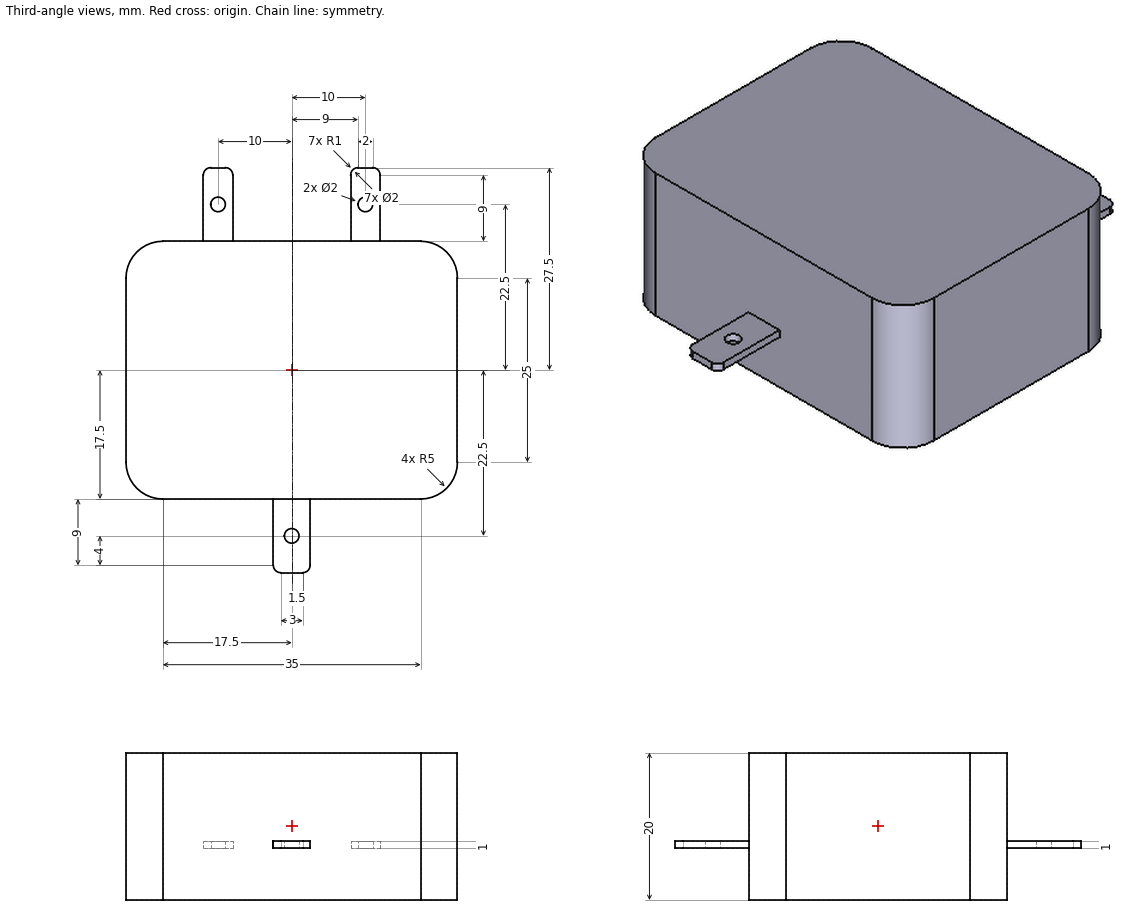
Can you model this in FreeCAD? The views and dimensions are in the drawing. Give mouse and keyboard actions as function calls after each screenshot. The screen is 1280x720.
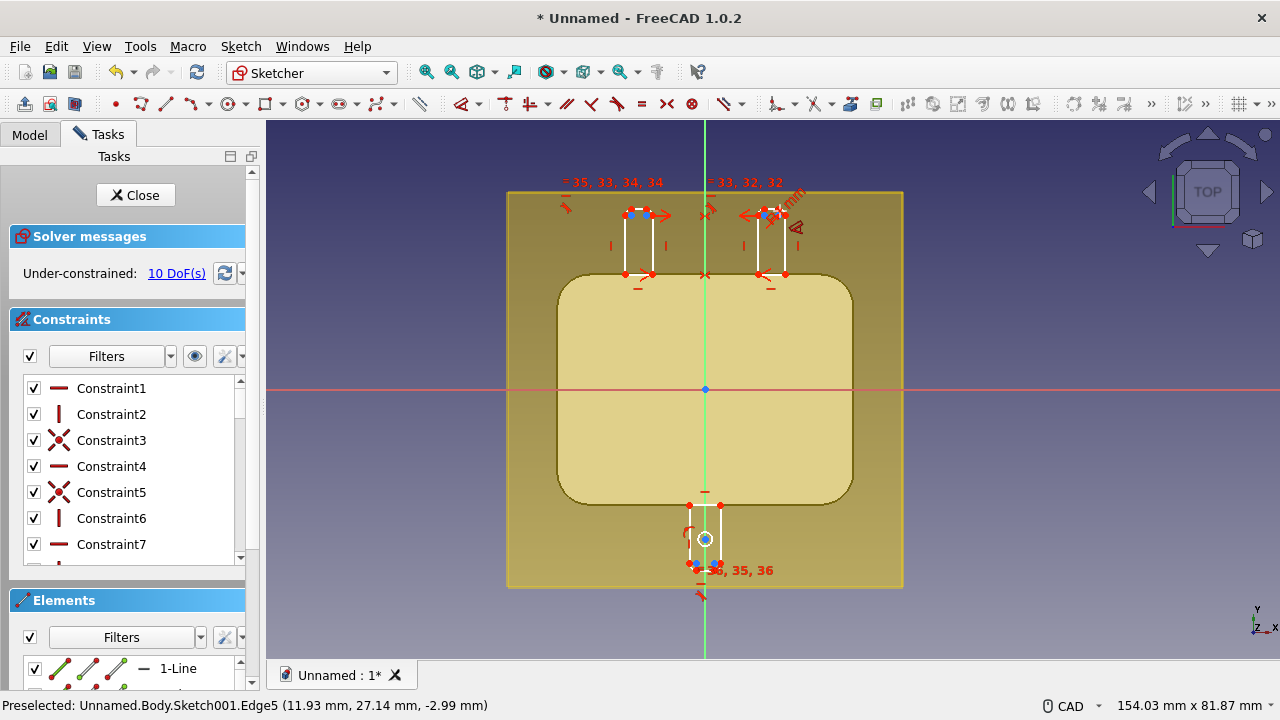
scroll(710, 534, up, 6)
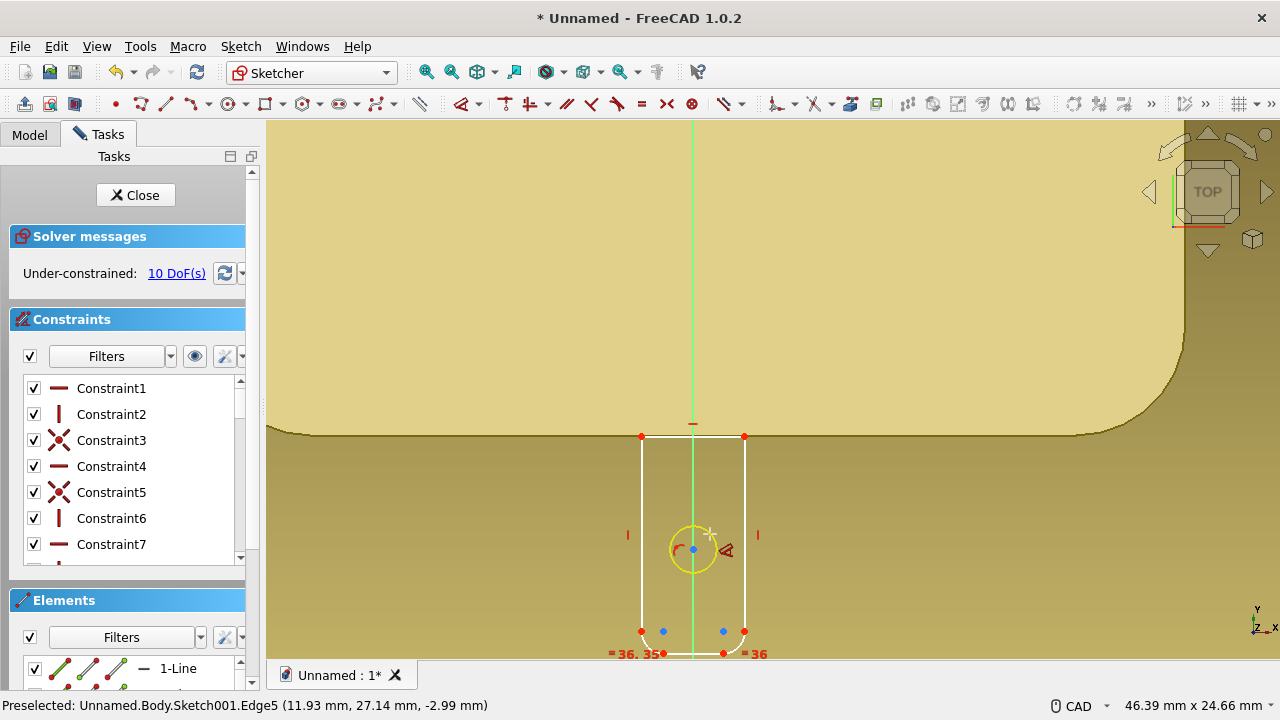
click(710, 533)
click(709, 496)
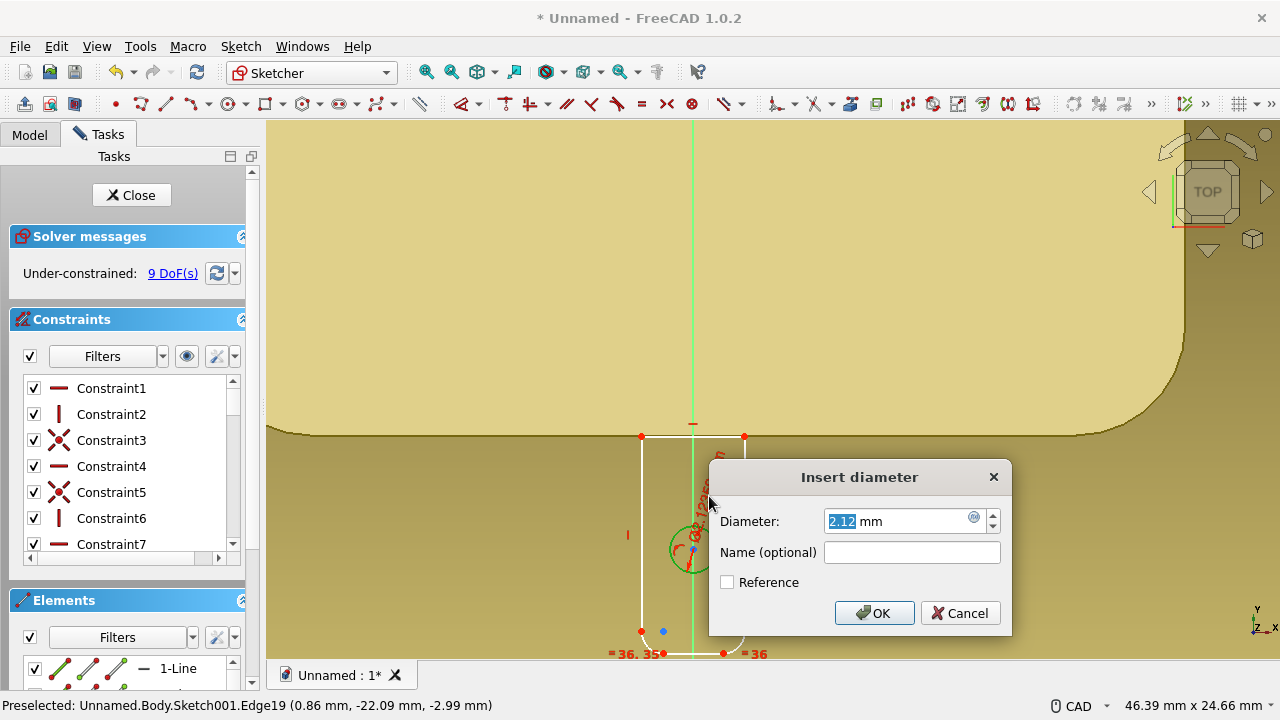
text(2)
key(Return)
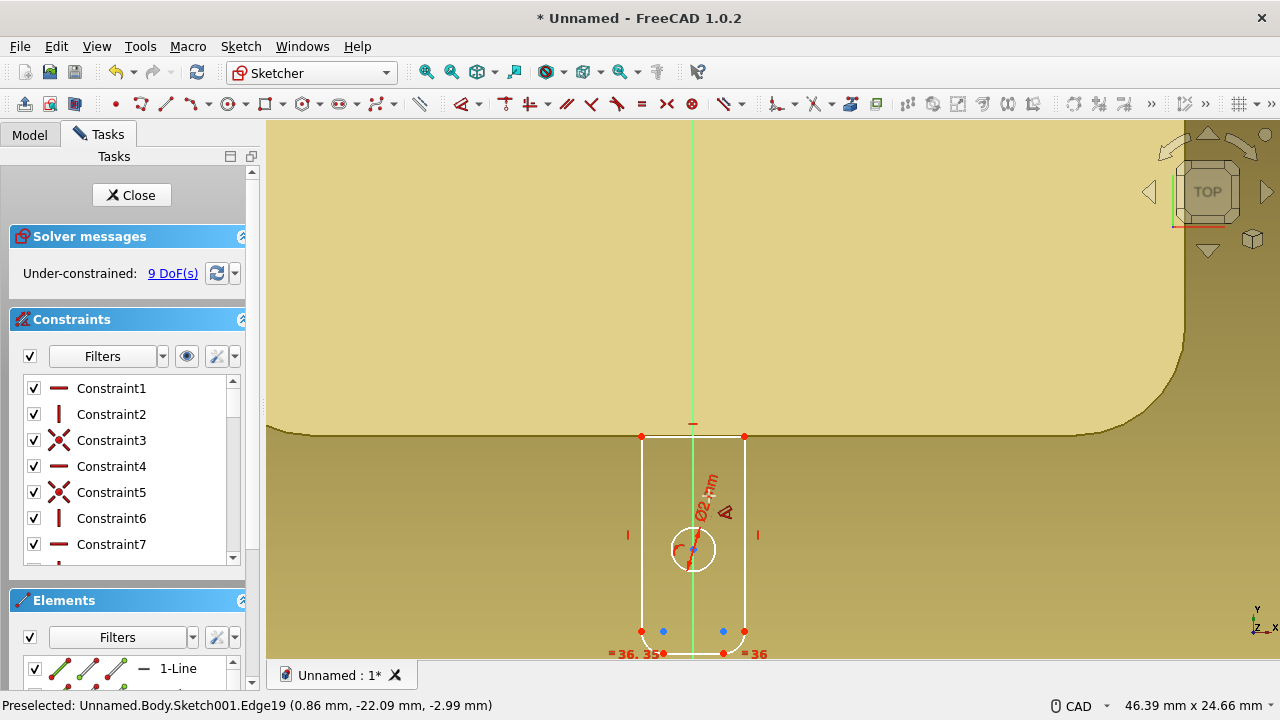
scroll(709, 535, down, 6)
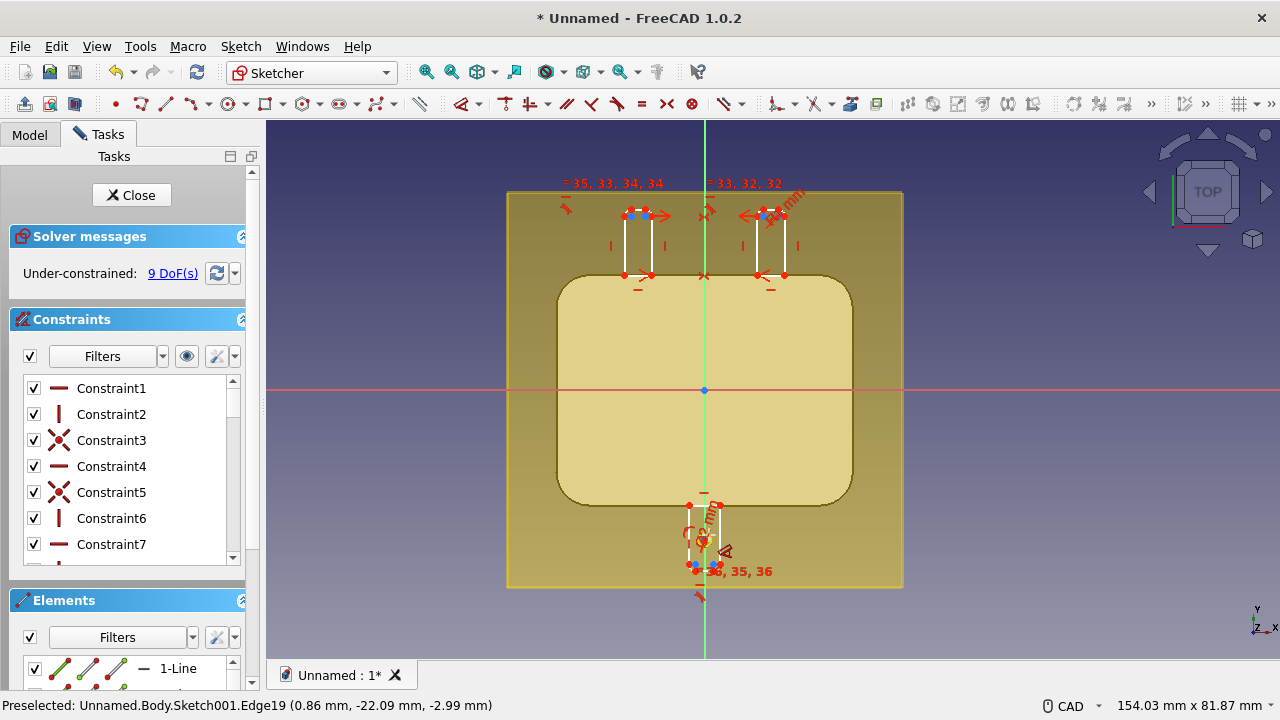
scroll(768, 210, up, 6)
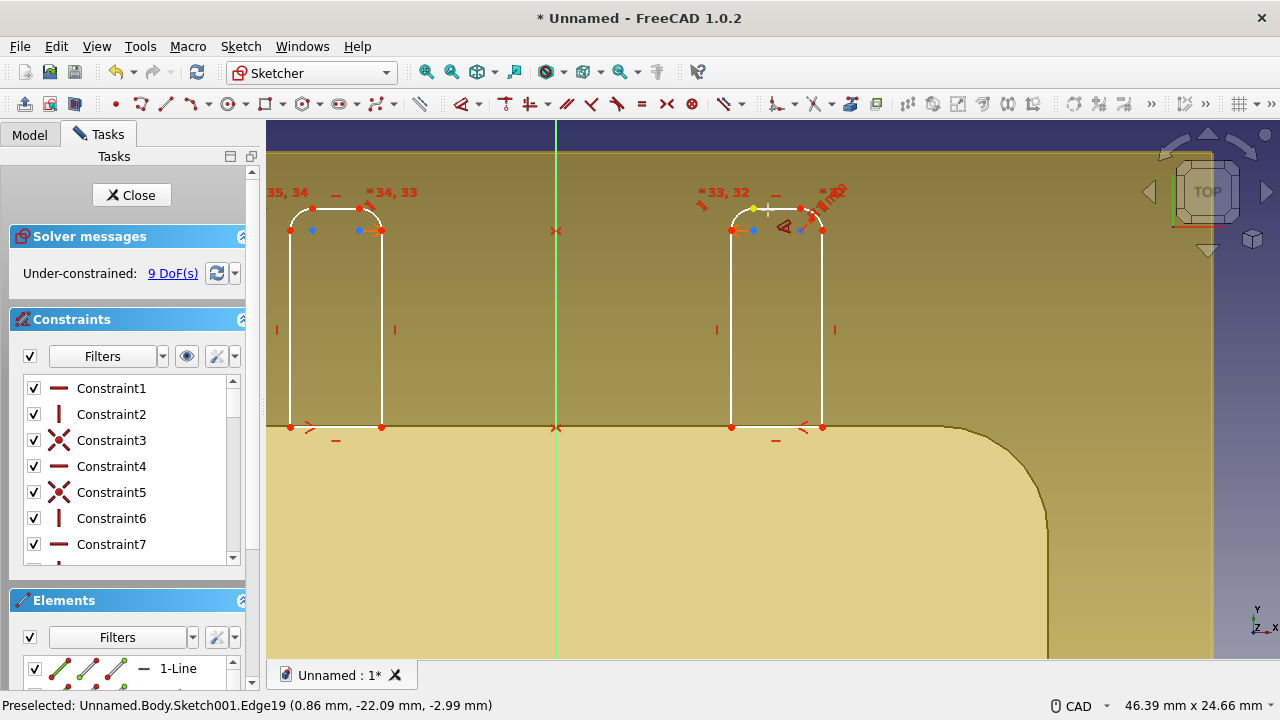
click(767, 209)
click(777, 175)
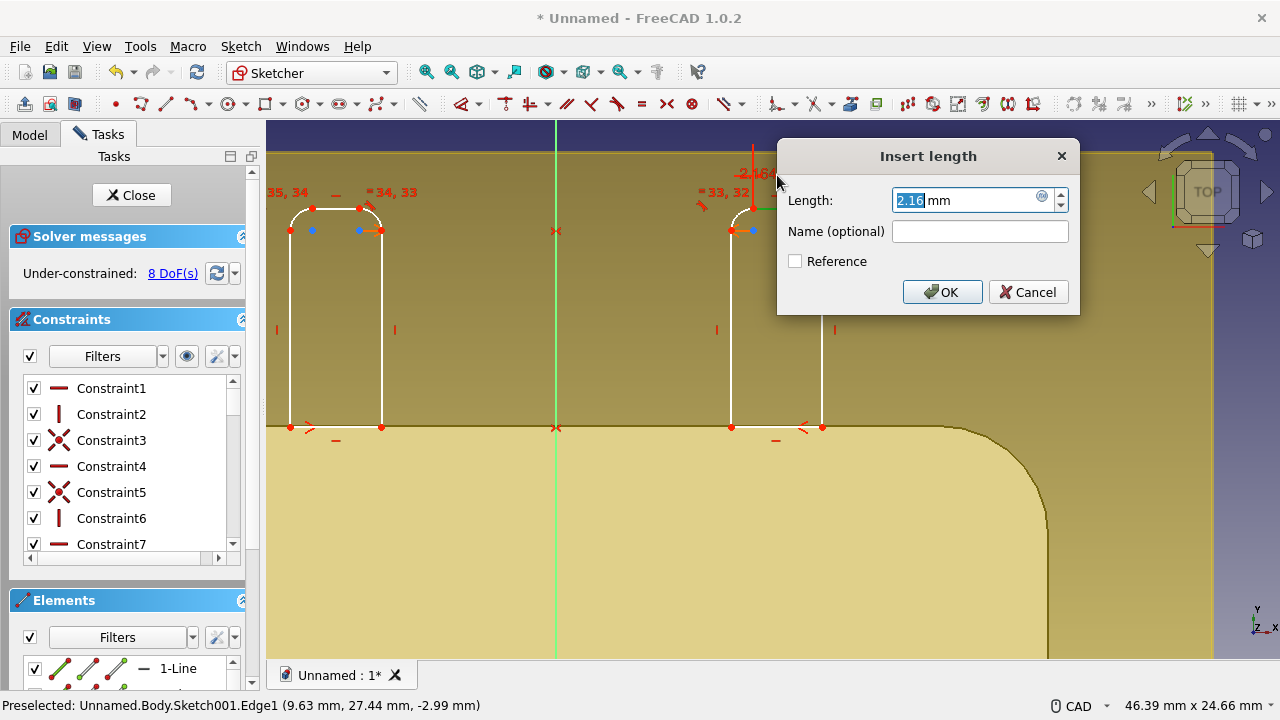
text(2)
key(Return)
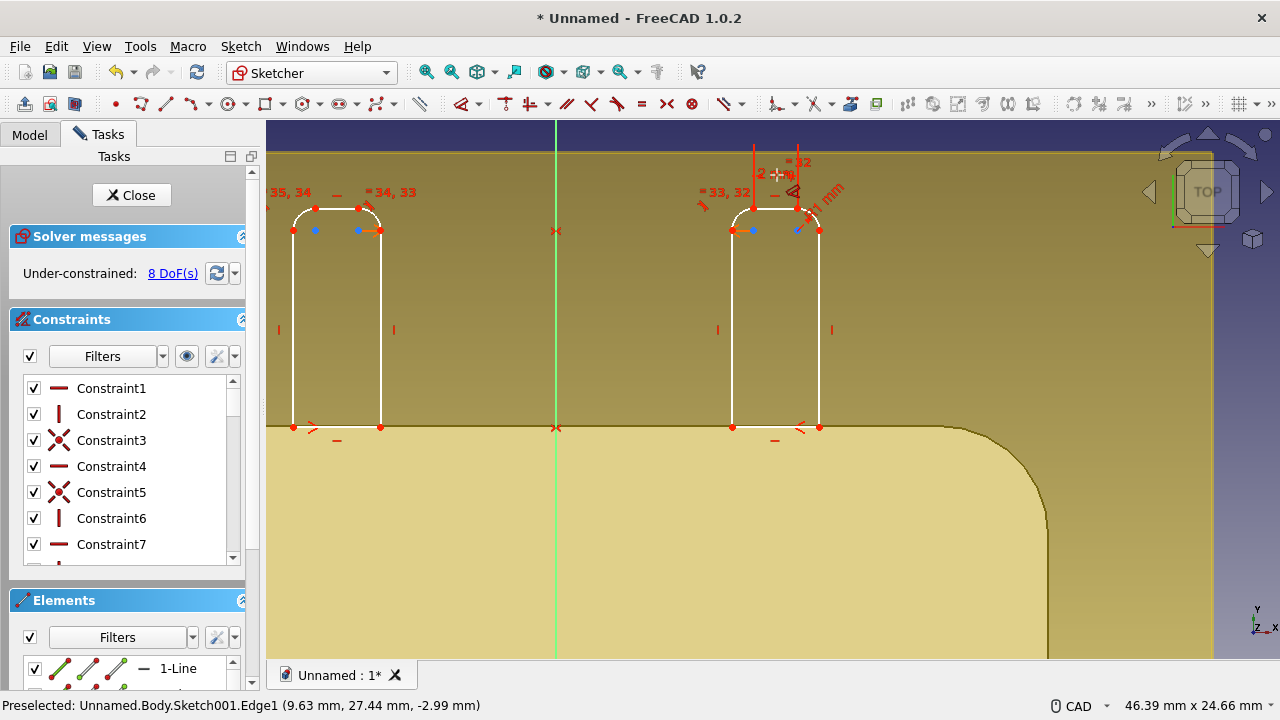
scroll(768, 209, down, 6)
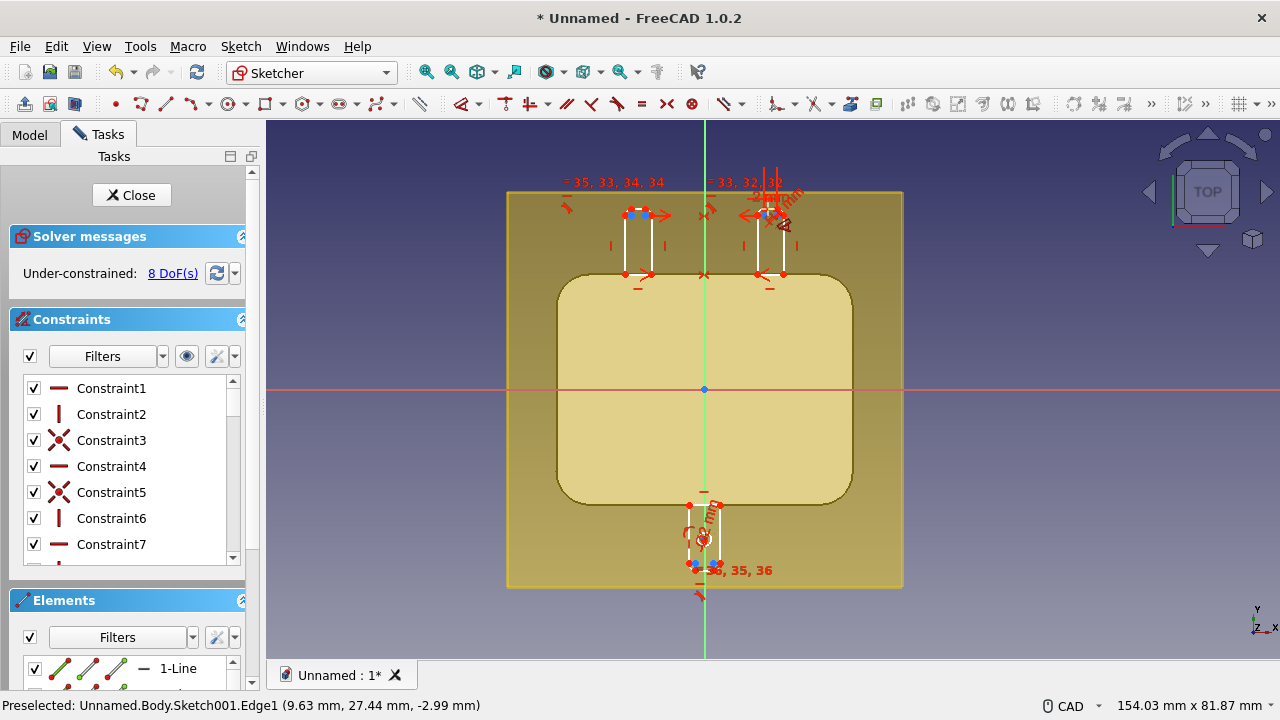
click(784, 233)
click(818, 245)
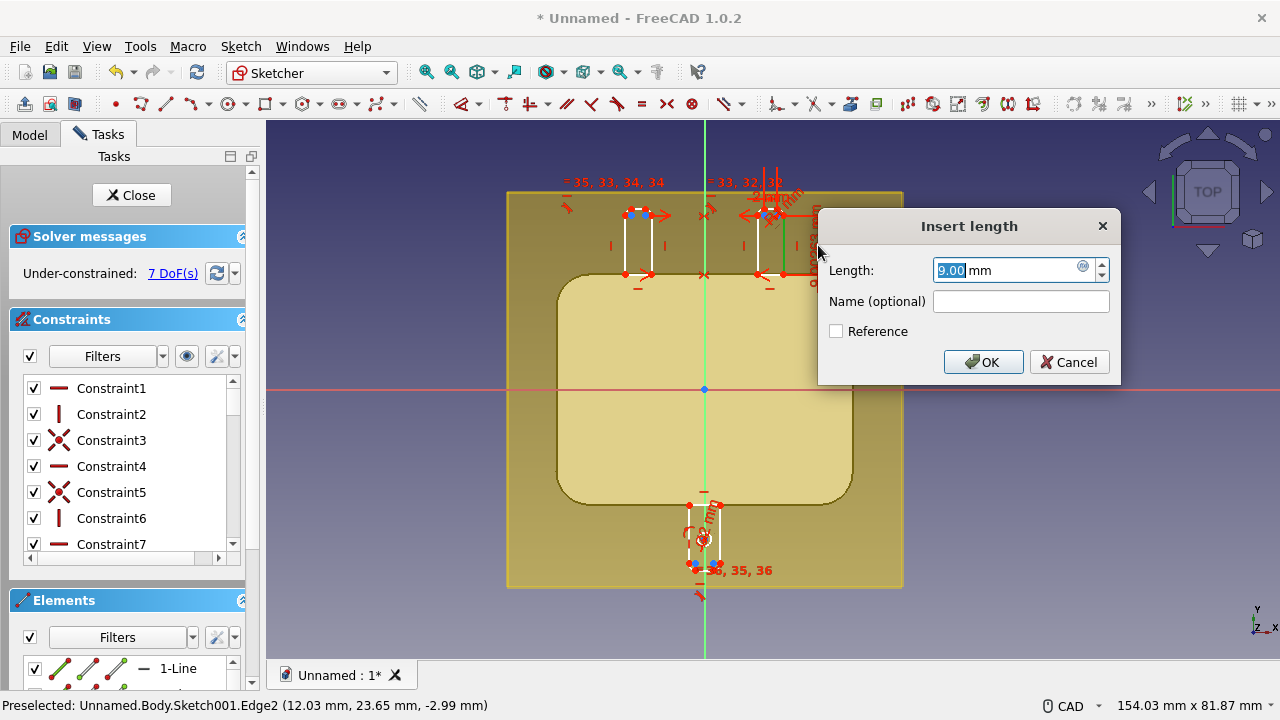
text(9)
key(Return)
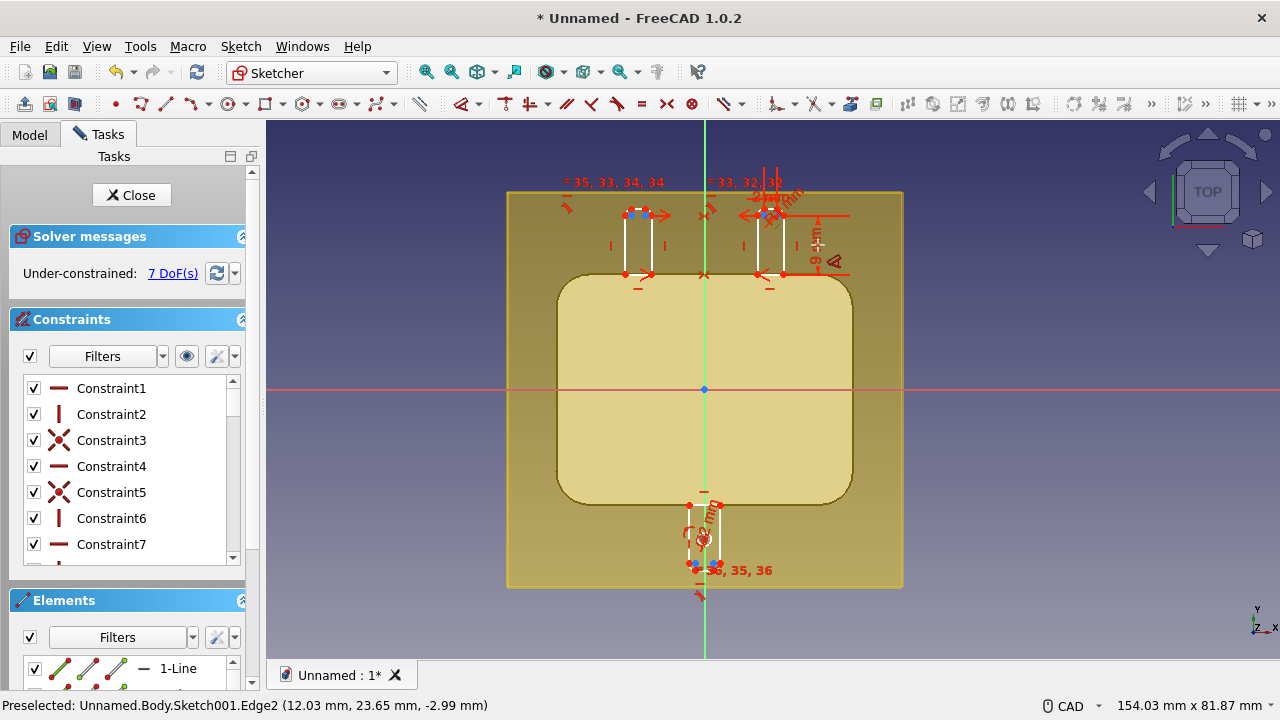
scroll(705, 571, up, 4)